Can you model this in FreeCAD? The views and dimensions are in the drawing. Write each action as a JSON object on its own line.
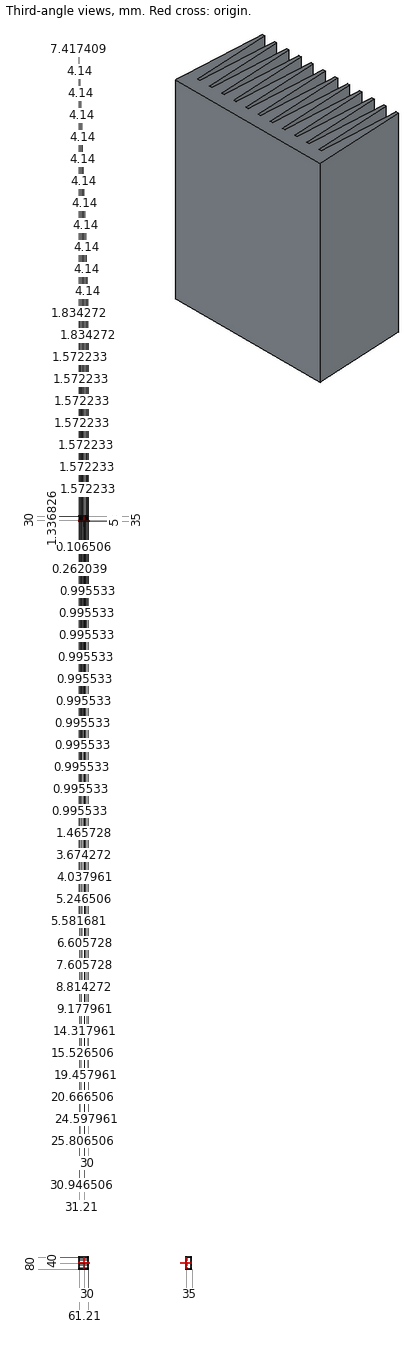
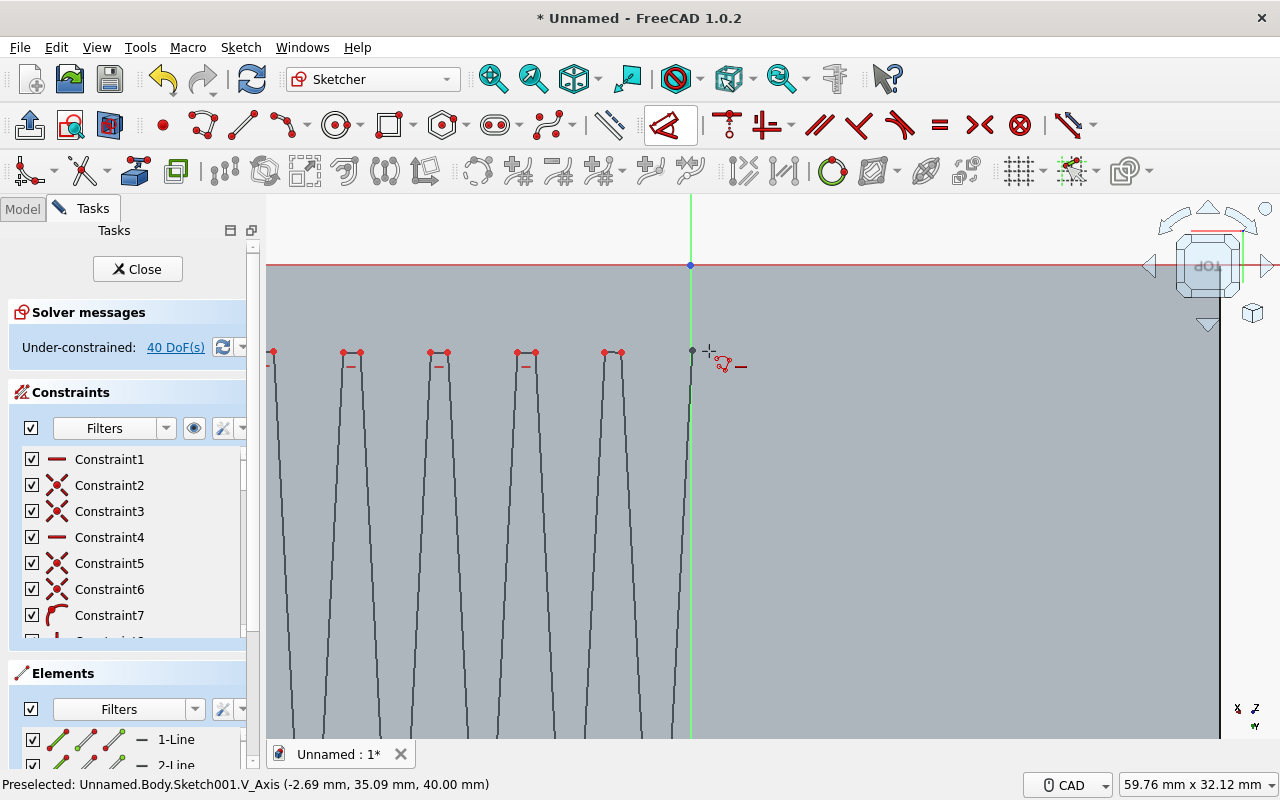
{"action": "left_click", "coordinate": [709, 350]}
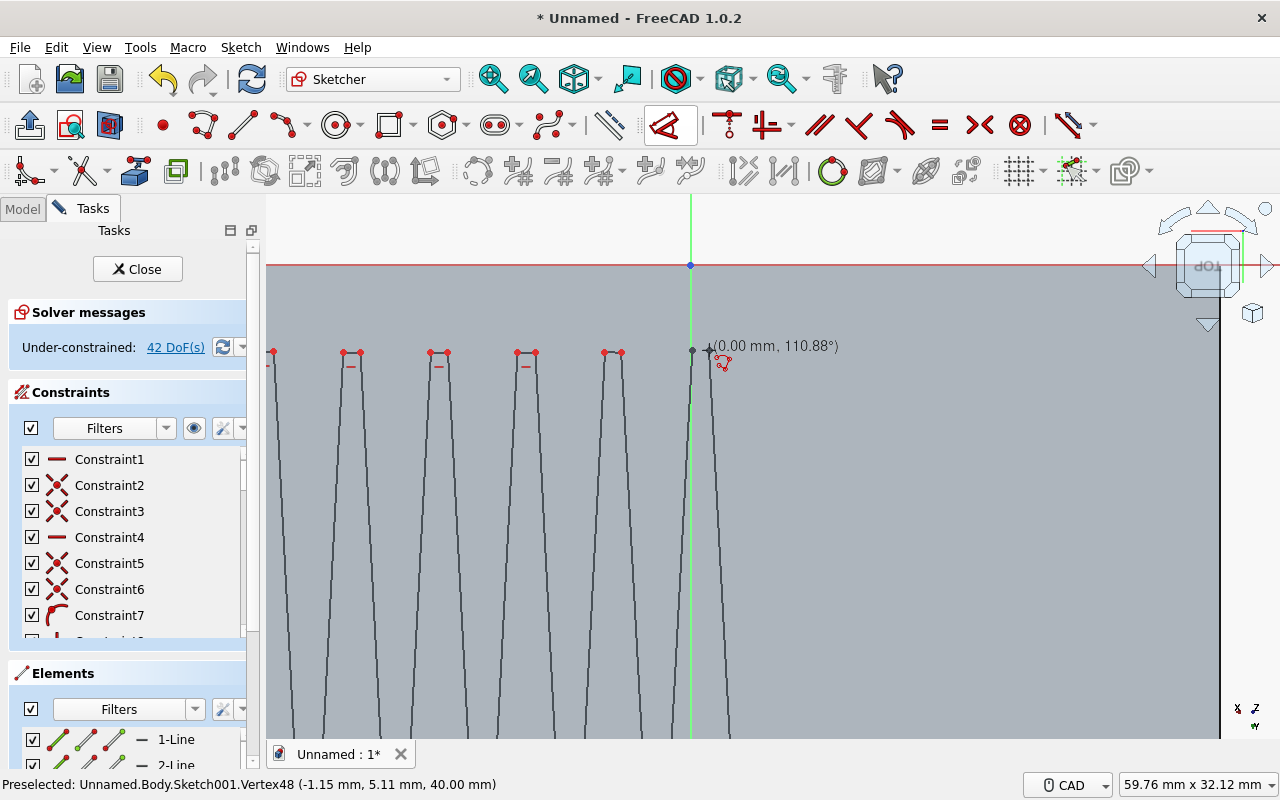
{"action": "scroll", "coordinate": [692, 350], "scroll_direction": "up", "scroll_amount": 11}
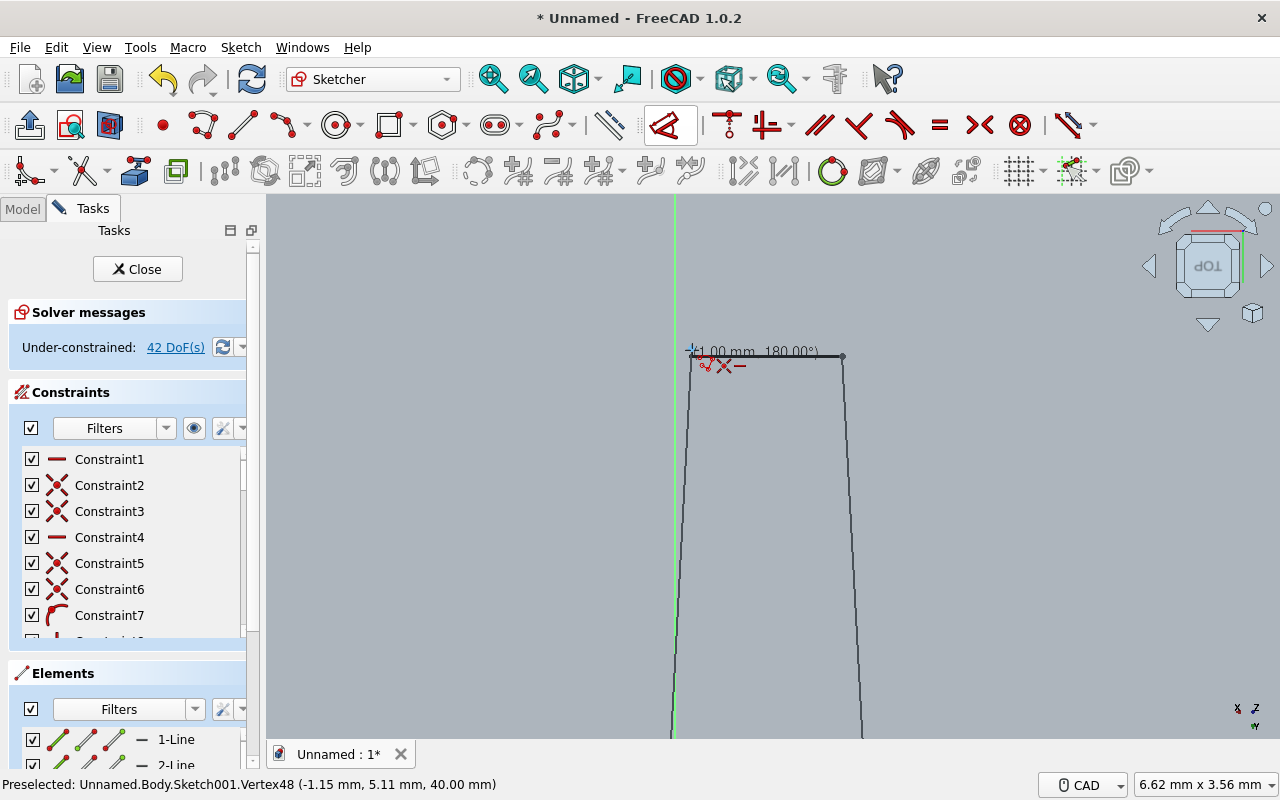
{"action": "left_click", "coordinate": [692, 349]}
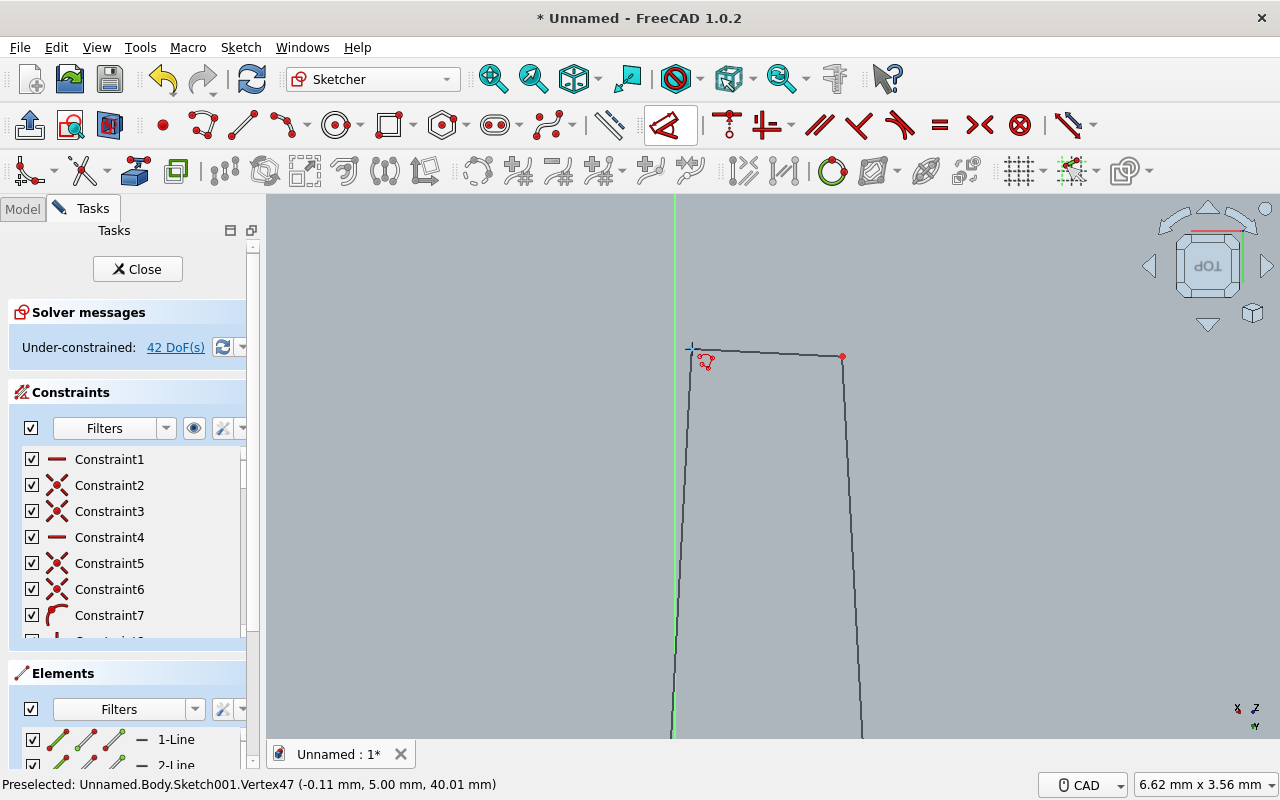
{"action": "scroll", "coordinate": [700, 350], "scroll_direction": "down", "scroll_amount": 14}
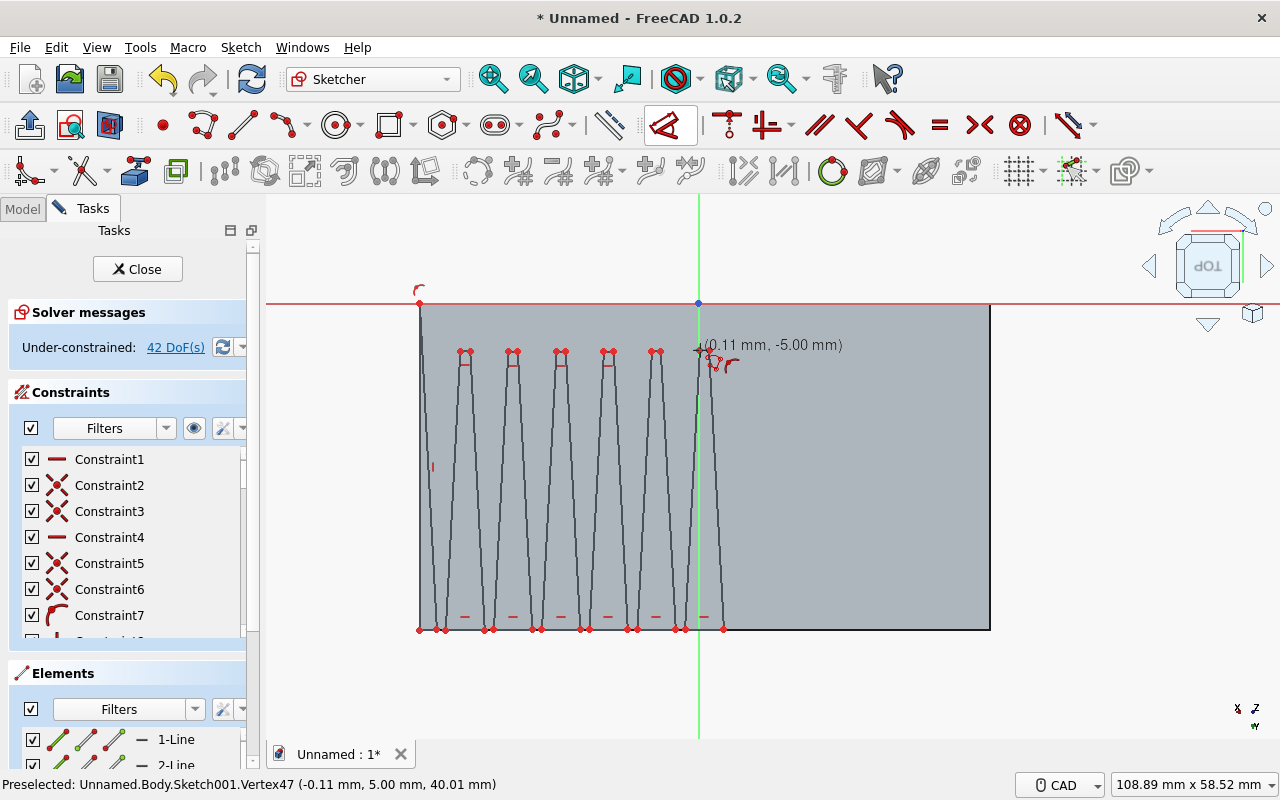
{"action": "left_click", "coordinate": [748, 350]}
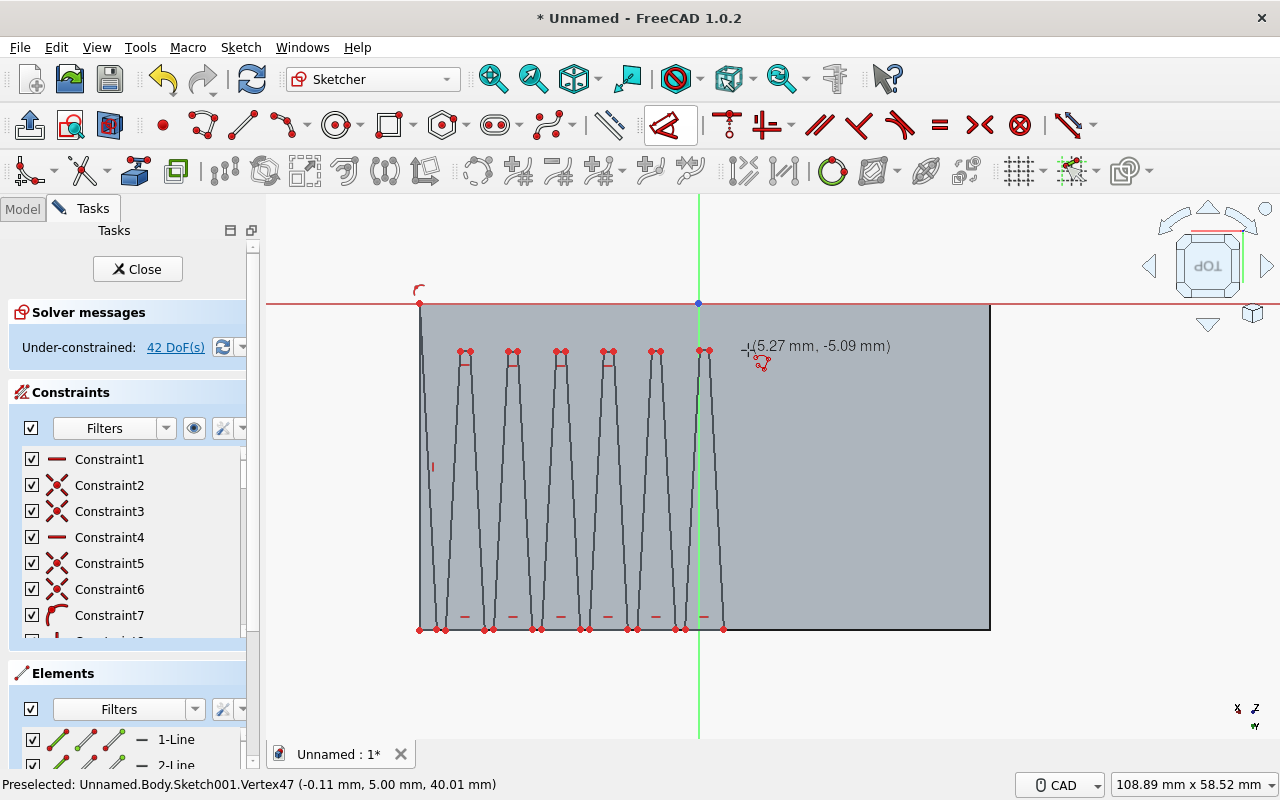
{"action": "scroll", "coordinate": [733, 630], "scroll_direction": "up", "scroll_amount": 3}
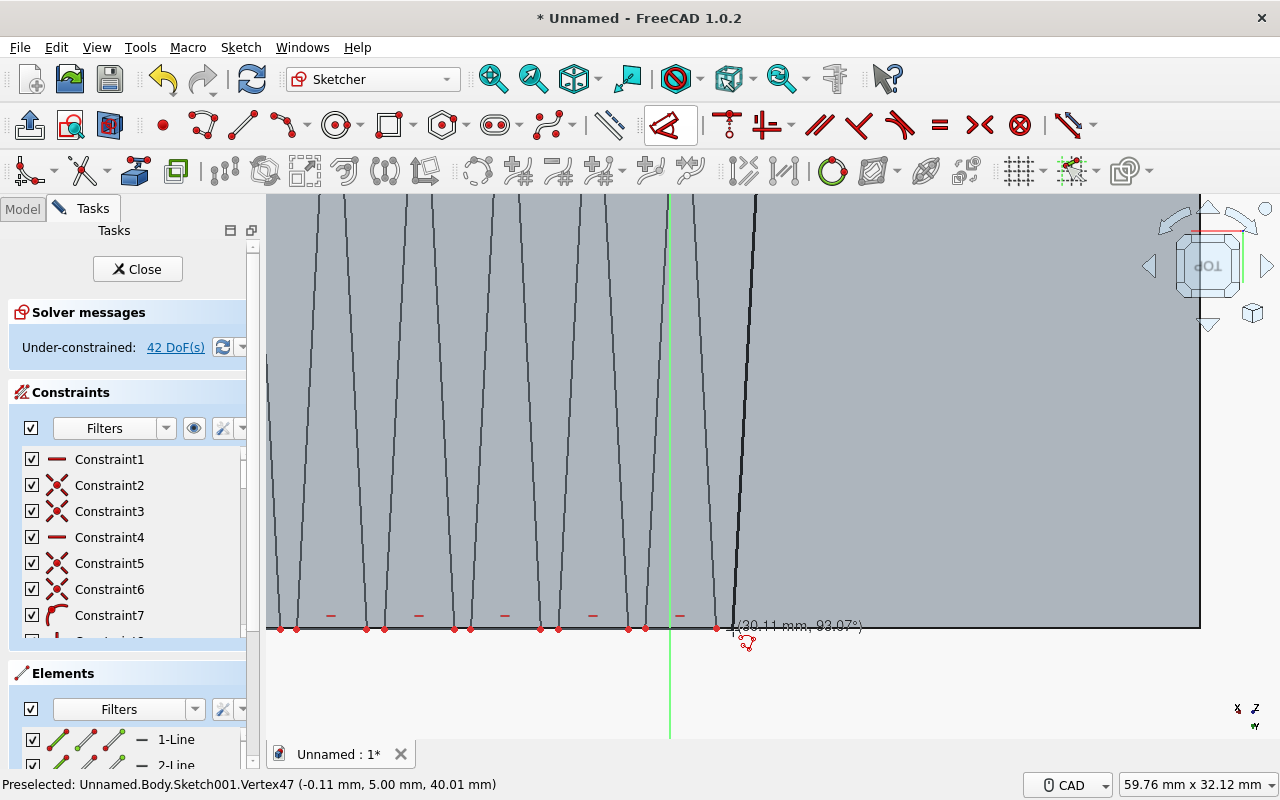
{"action": "left_click", "coordinate": [733, 628]}
{"action": "left_click", "coordinate": [803, 628]}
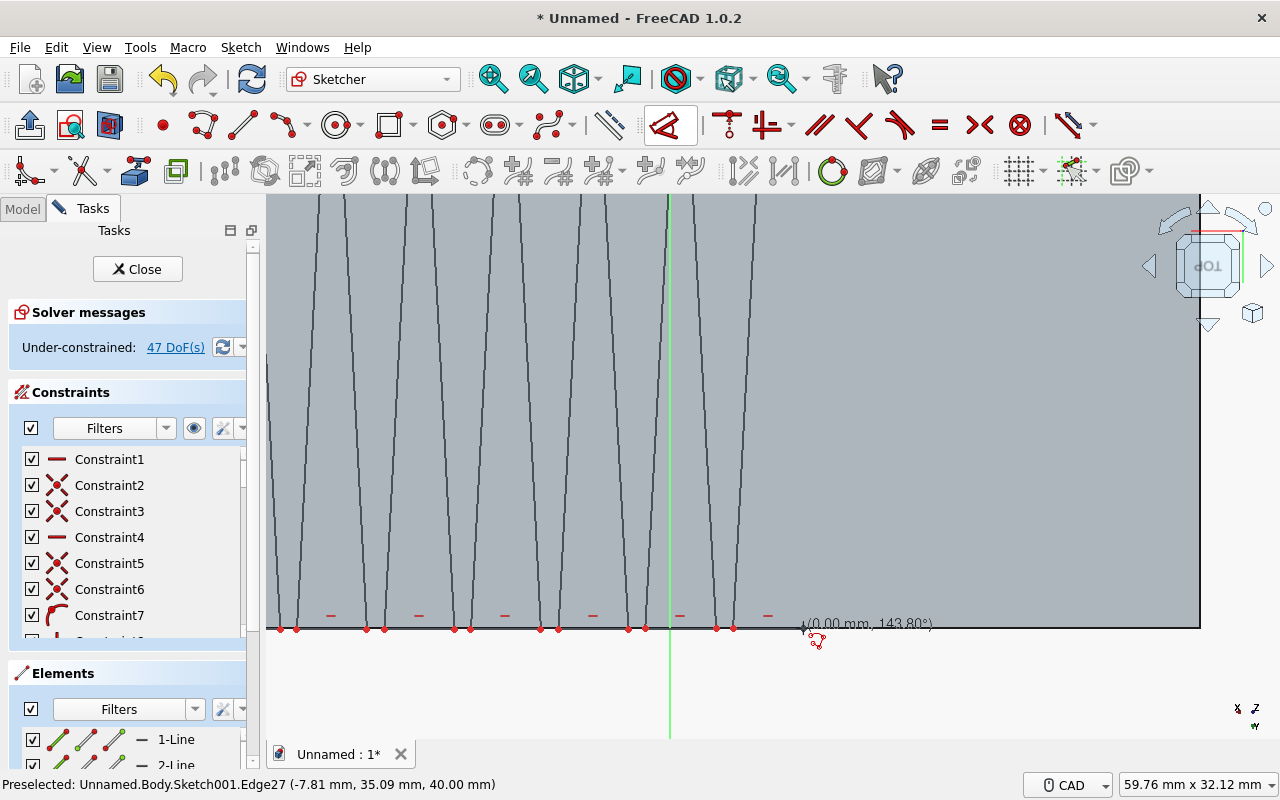
{"action": "scroll", "coordinate": [733, 631], "scroll_direction": "down", "scroll_amount": 3}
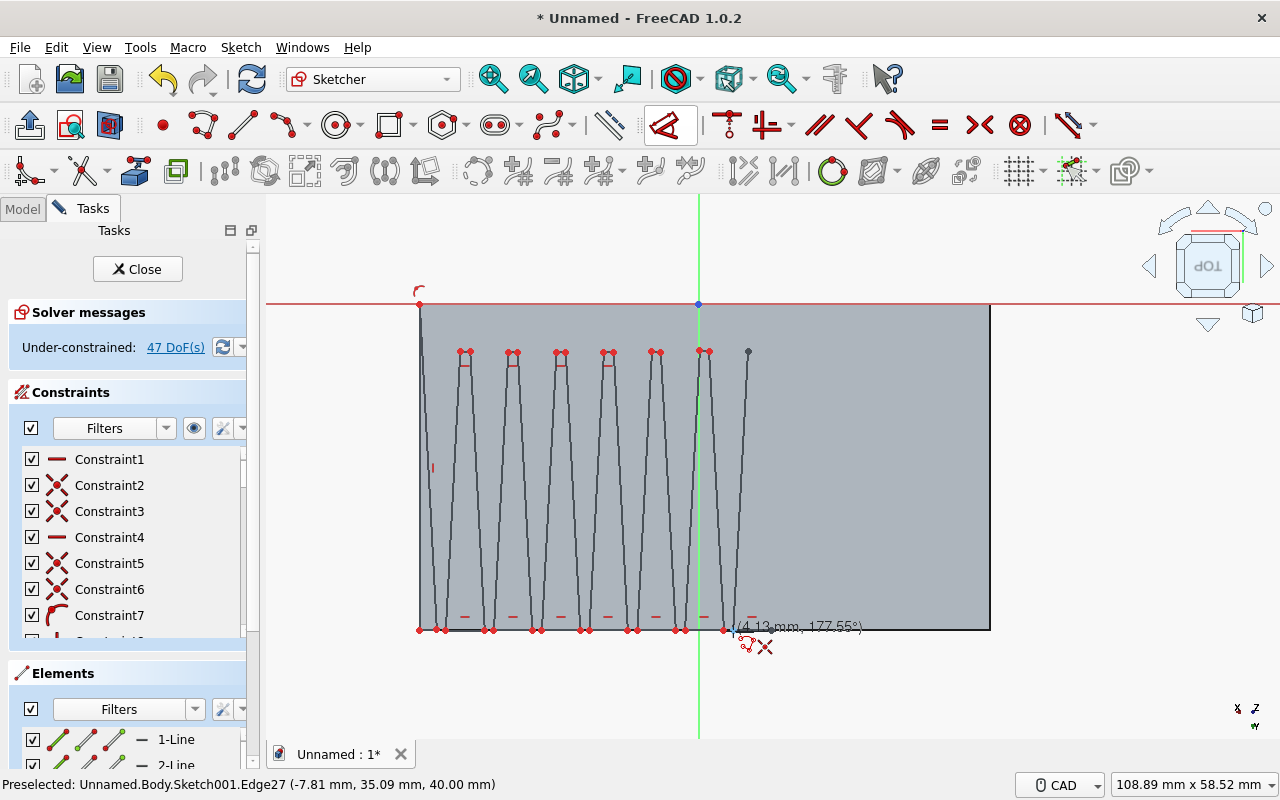
{"action": "scroll", "coordinate": [757, 351], "scroll_direction": "up", "scroll_amount": 3}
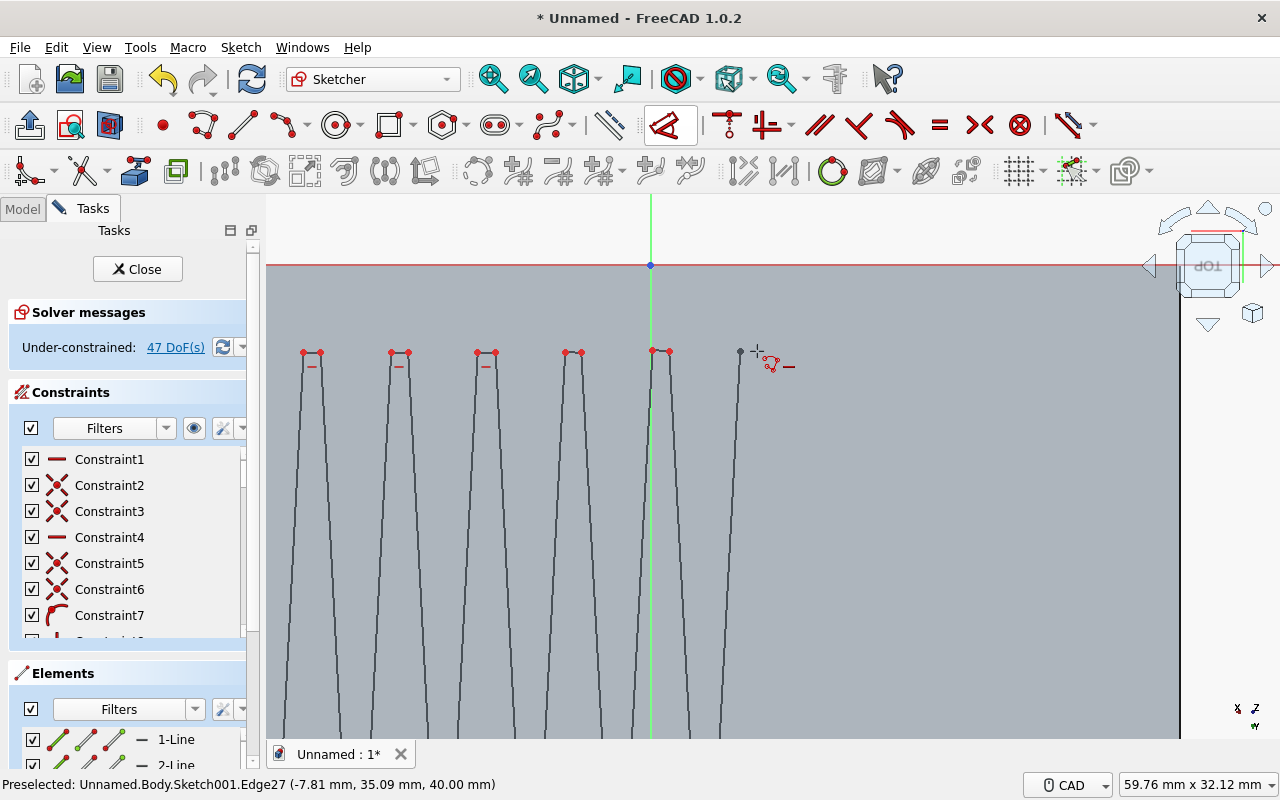
{"action": "left_click", "coordinate": [757, 350]}
{"action": "left_click", "coordinate": [740, 352]}